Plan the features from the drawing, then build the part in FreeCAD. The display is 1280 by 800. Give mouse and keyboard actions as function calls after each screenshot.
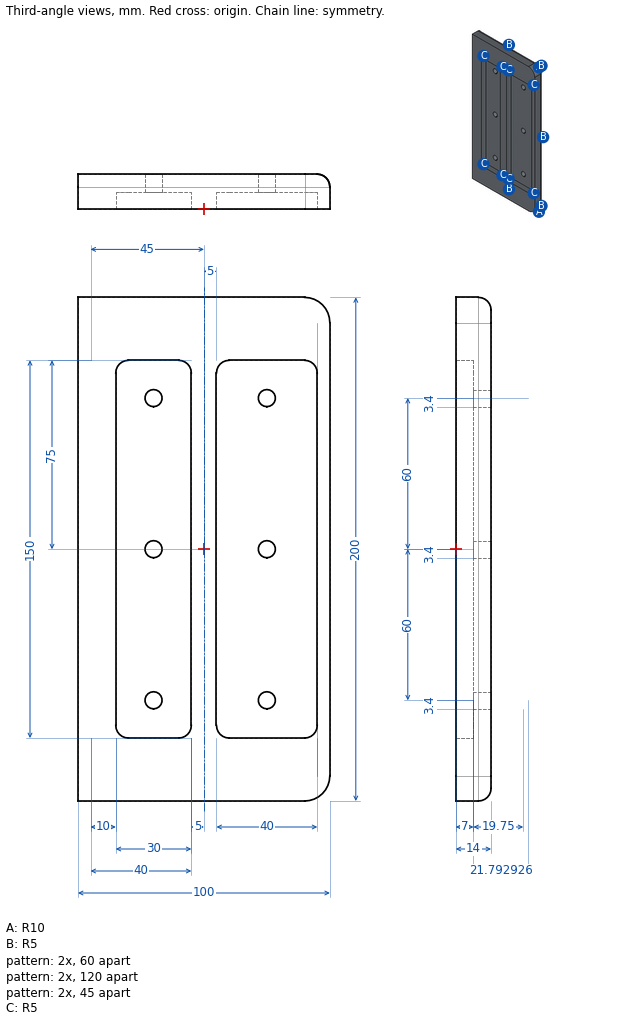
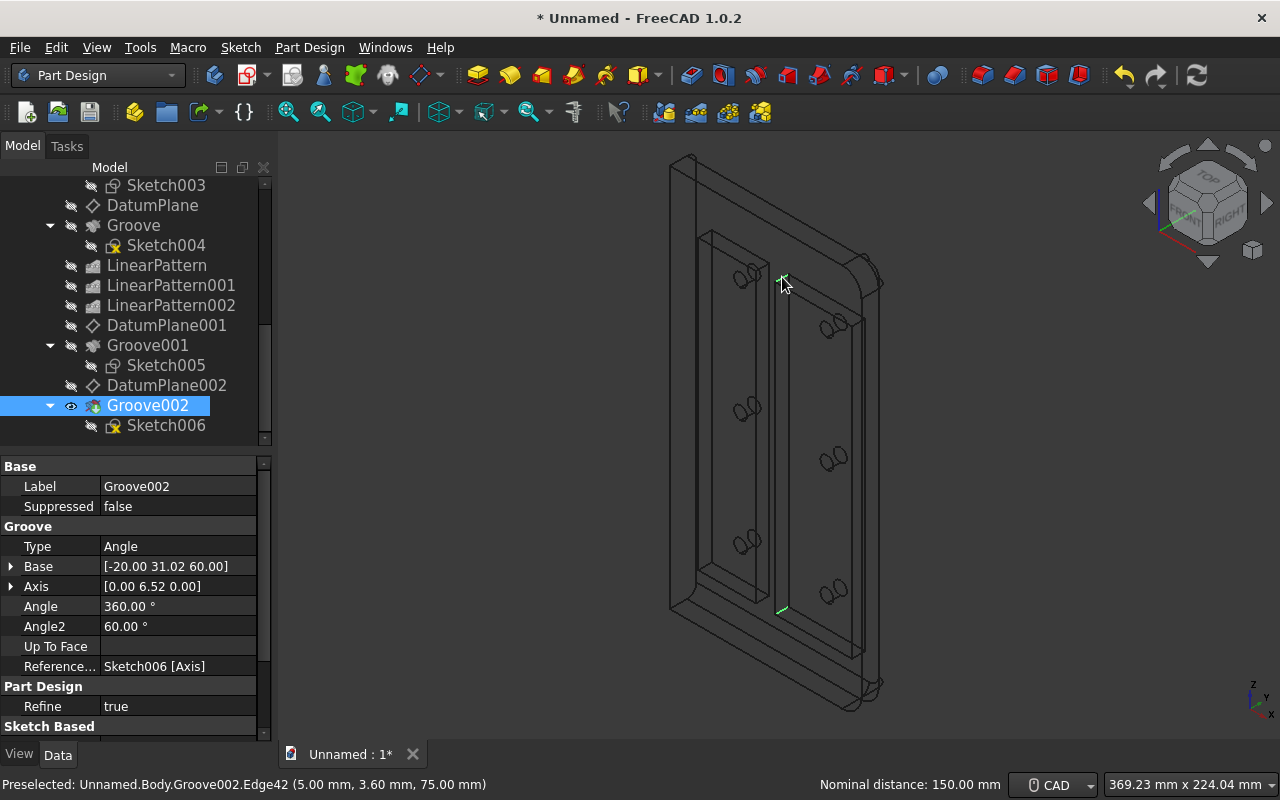
click(763, 266, ctrl)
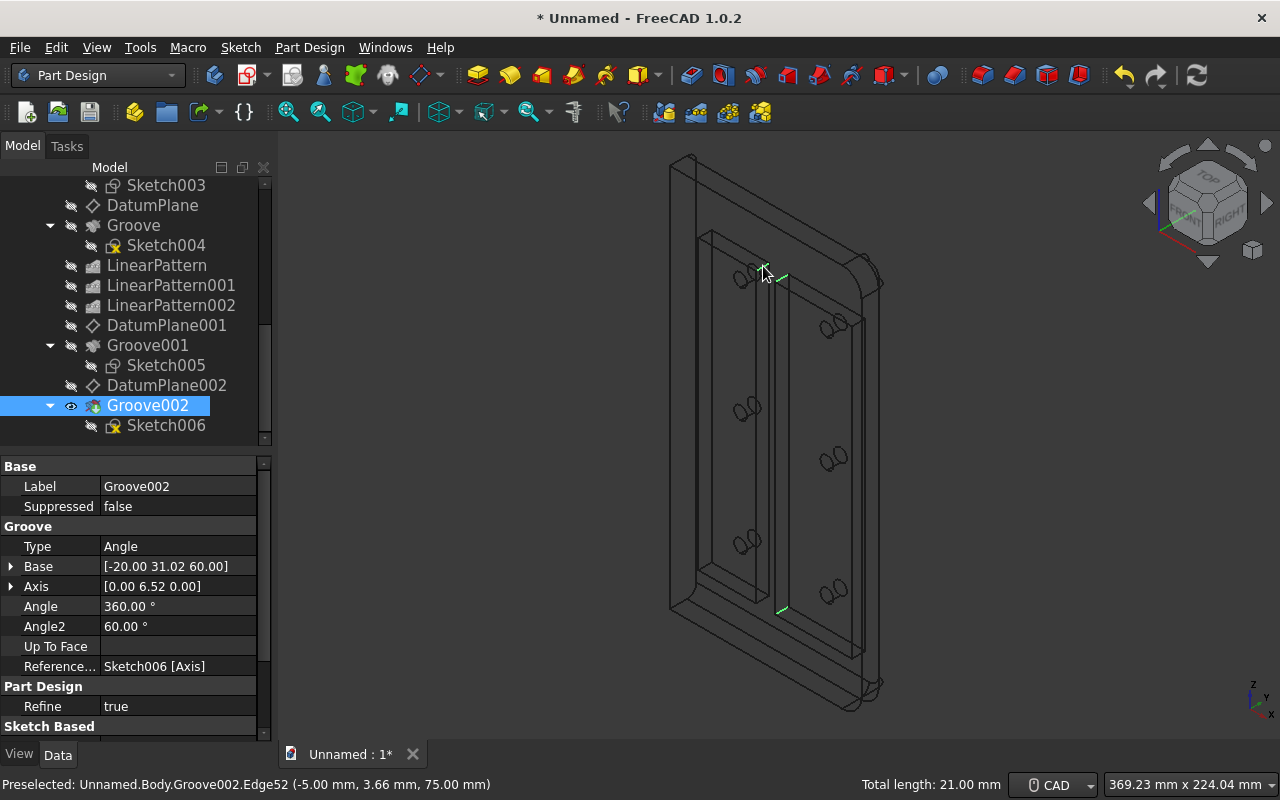
click(705, 565, ctrl)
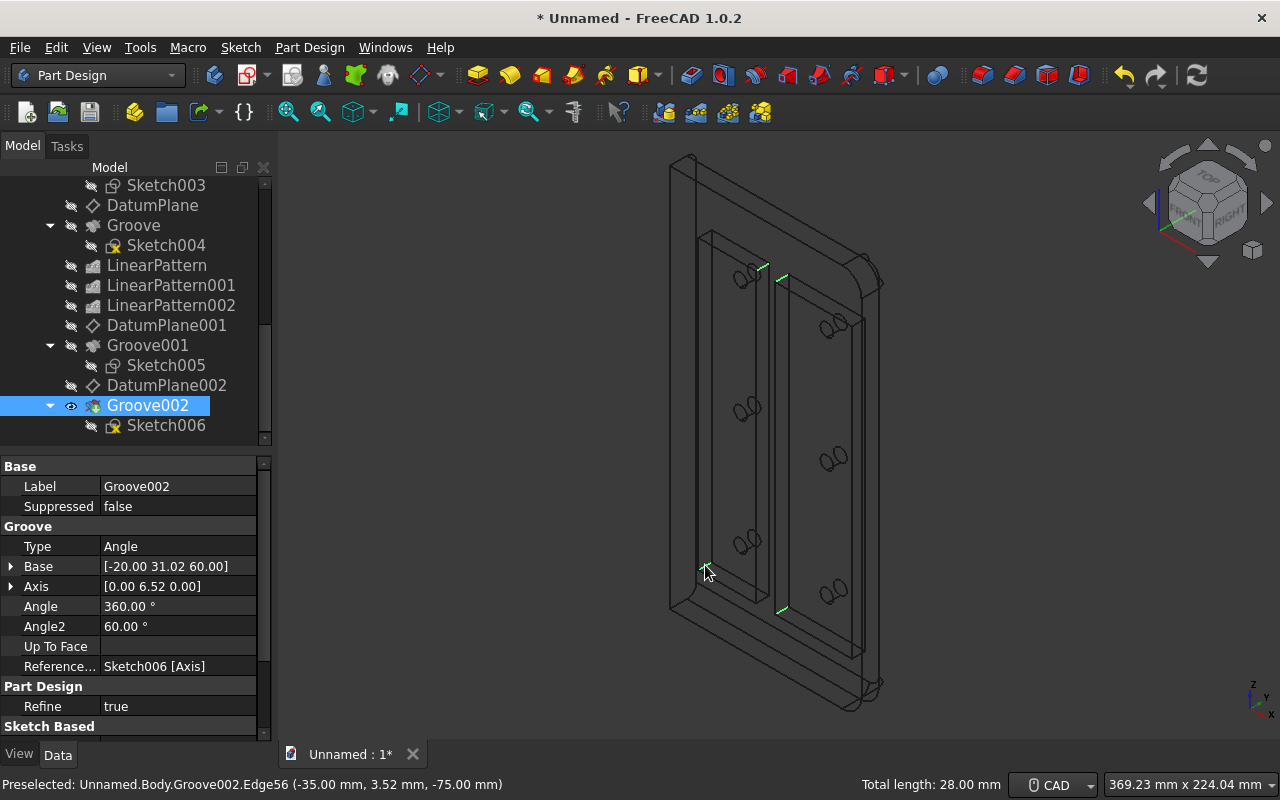
click(705, 233, ctrl)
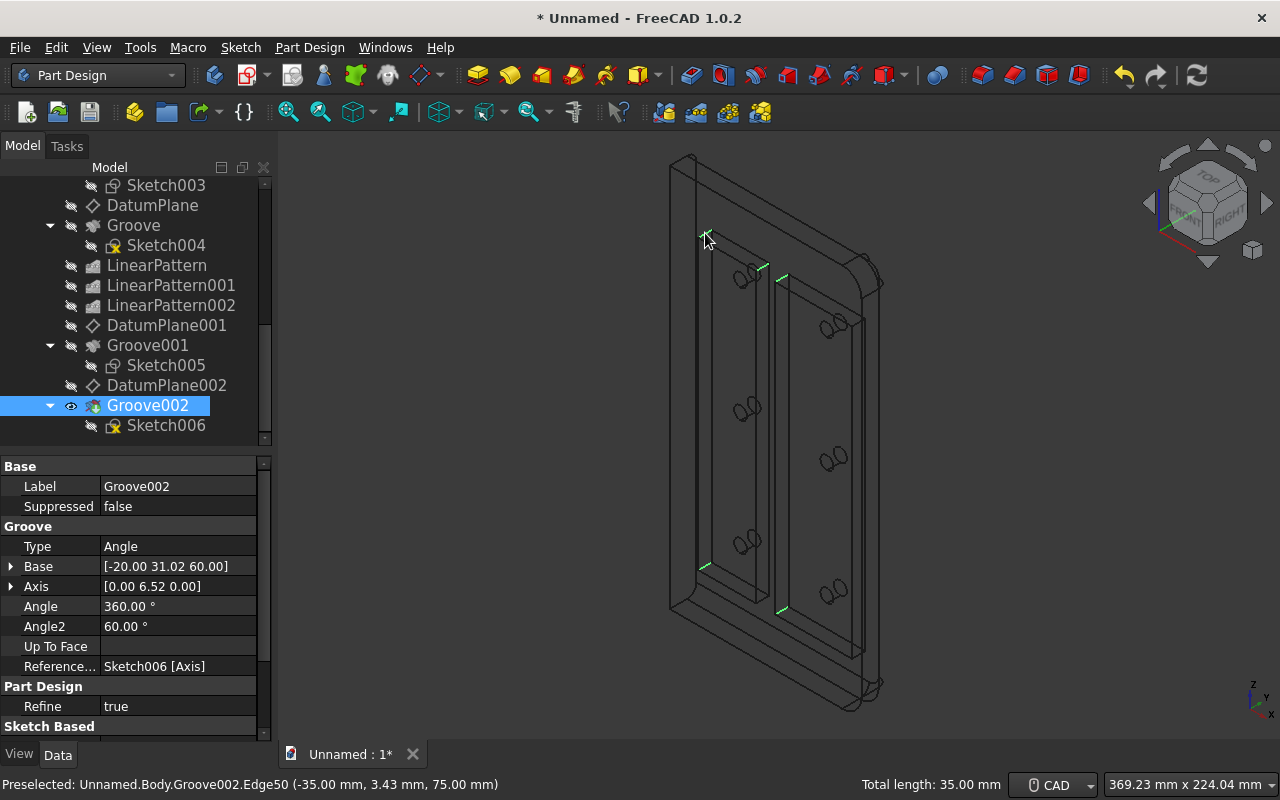
click(763, 599, ctrl)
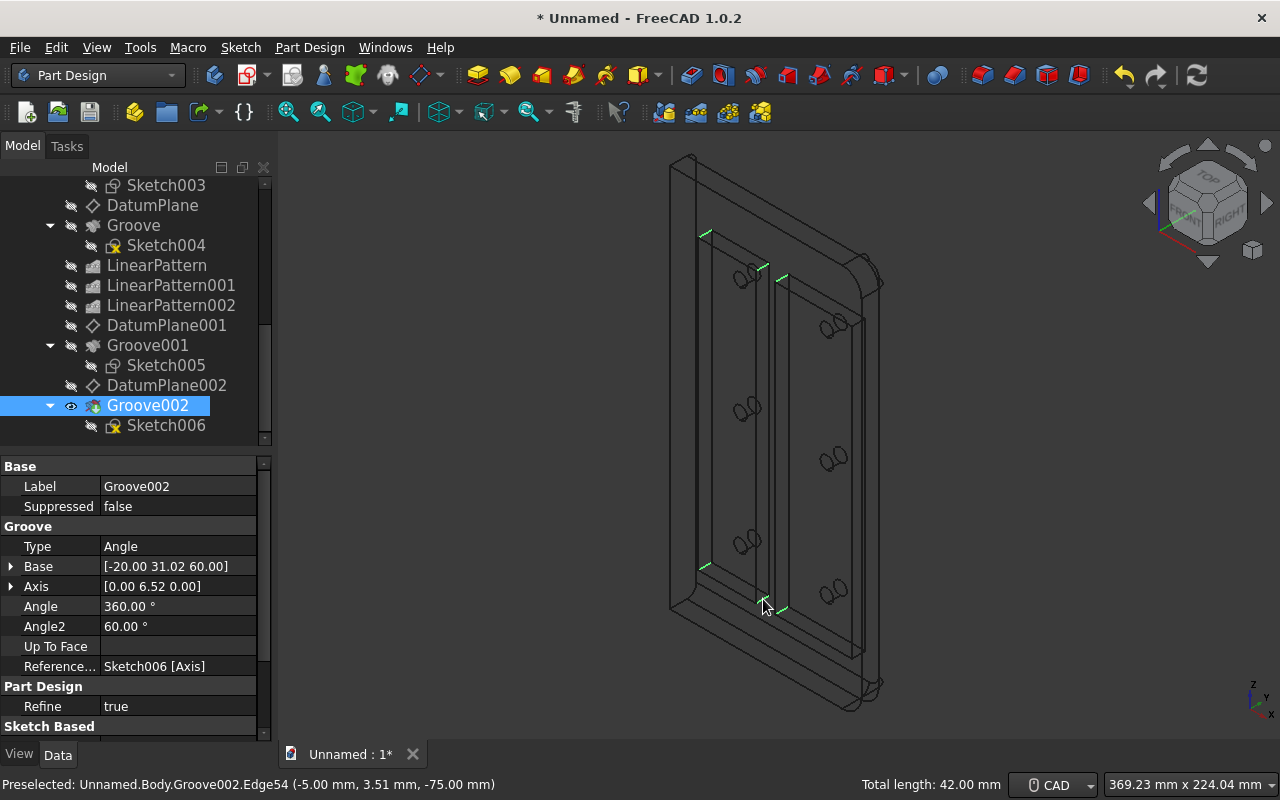
scroll(859, 322, up, 4)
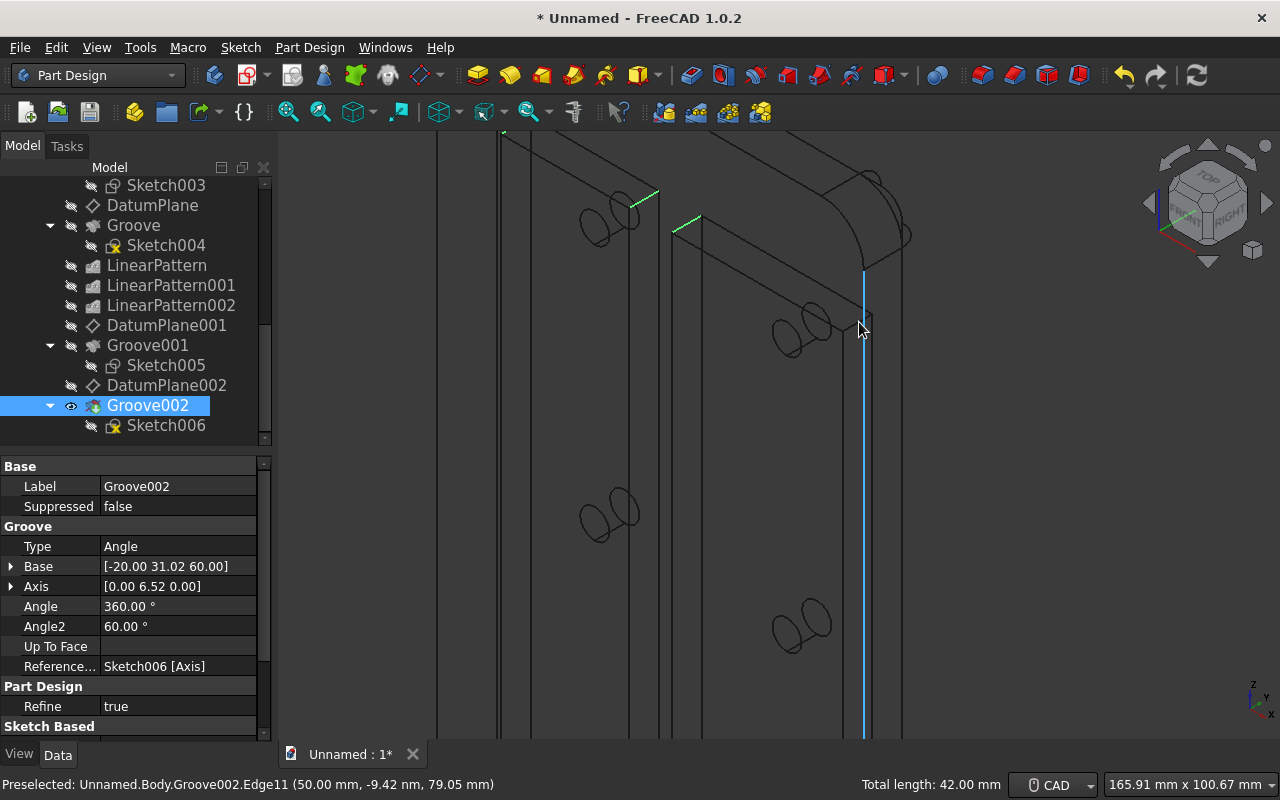
click(857, 322, ctrl)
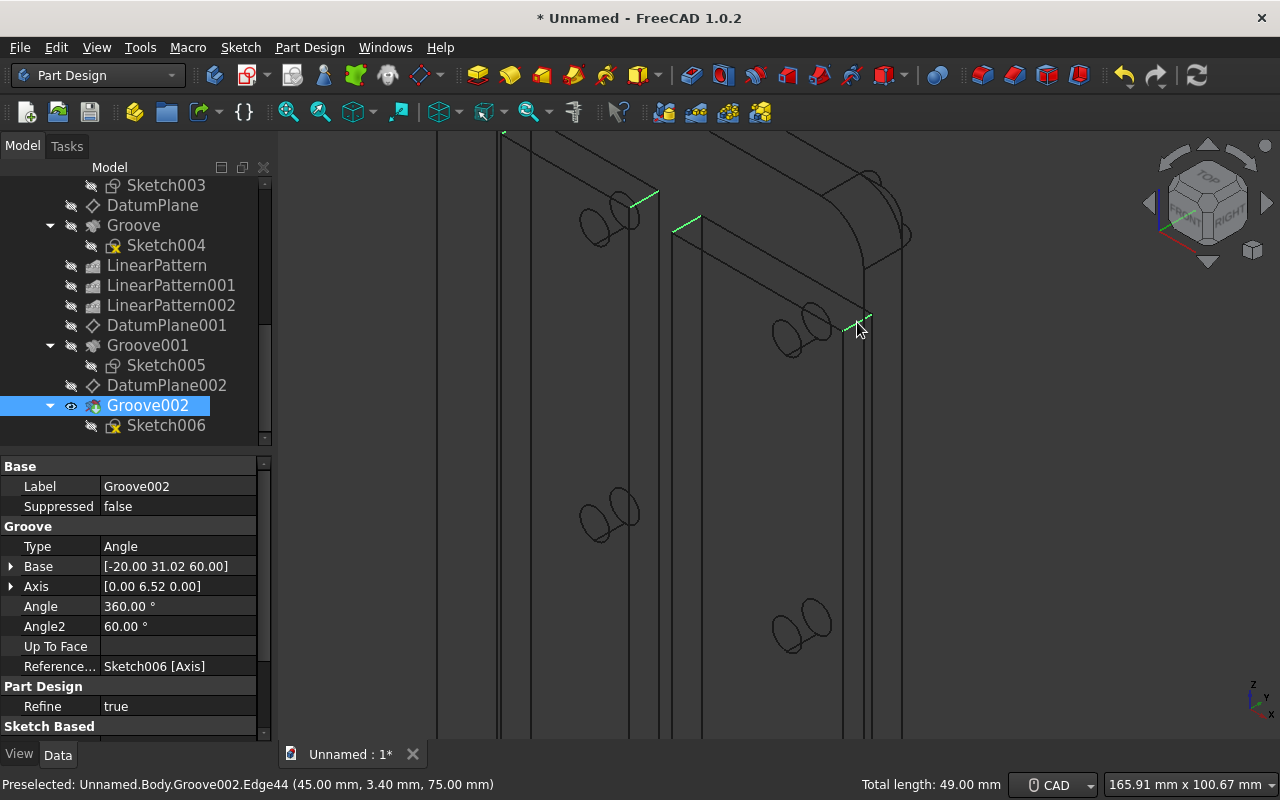
click(290, 112)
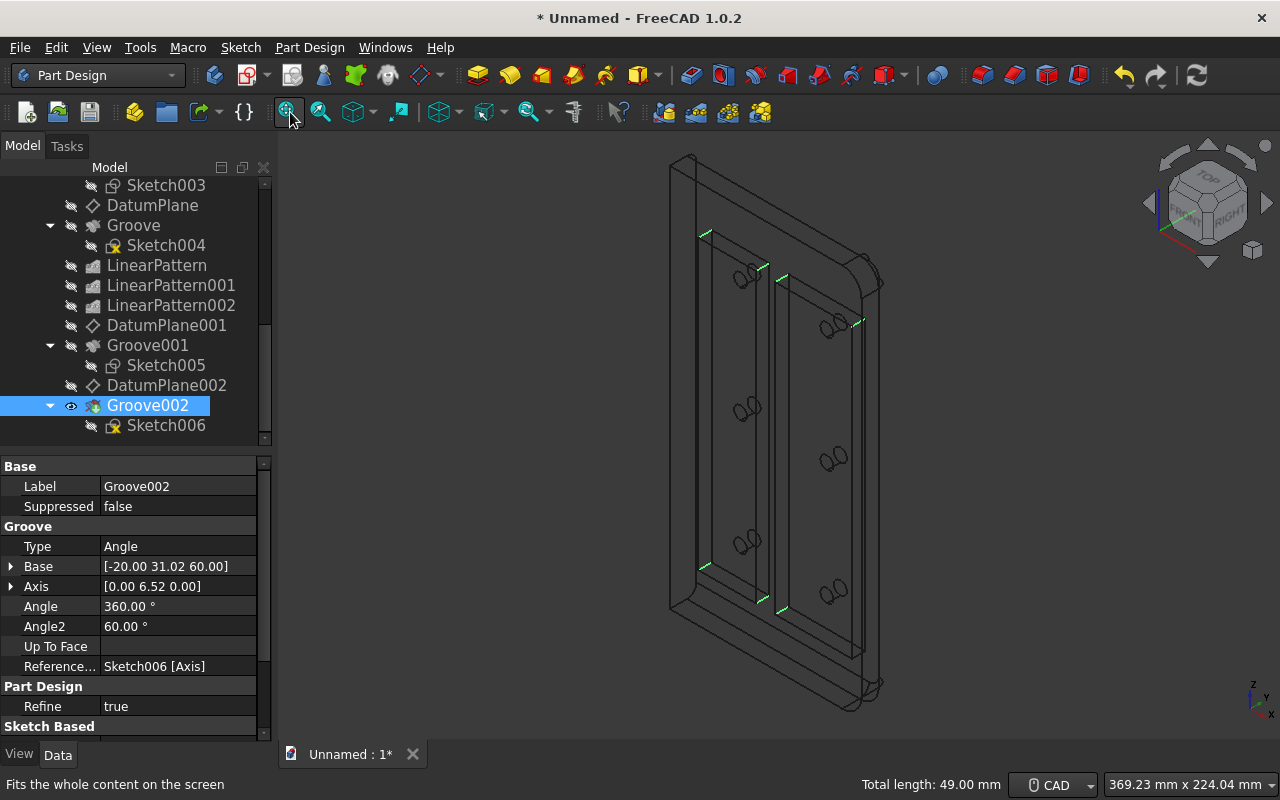
key(2)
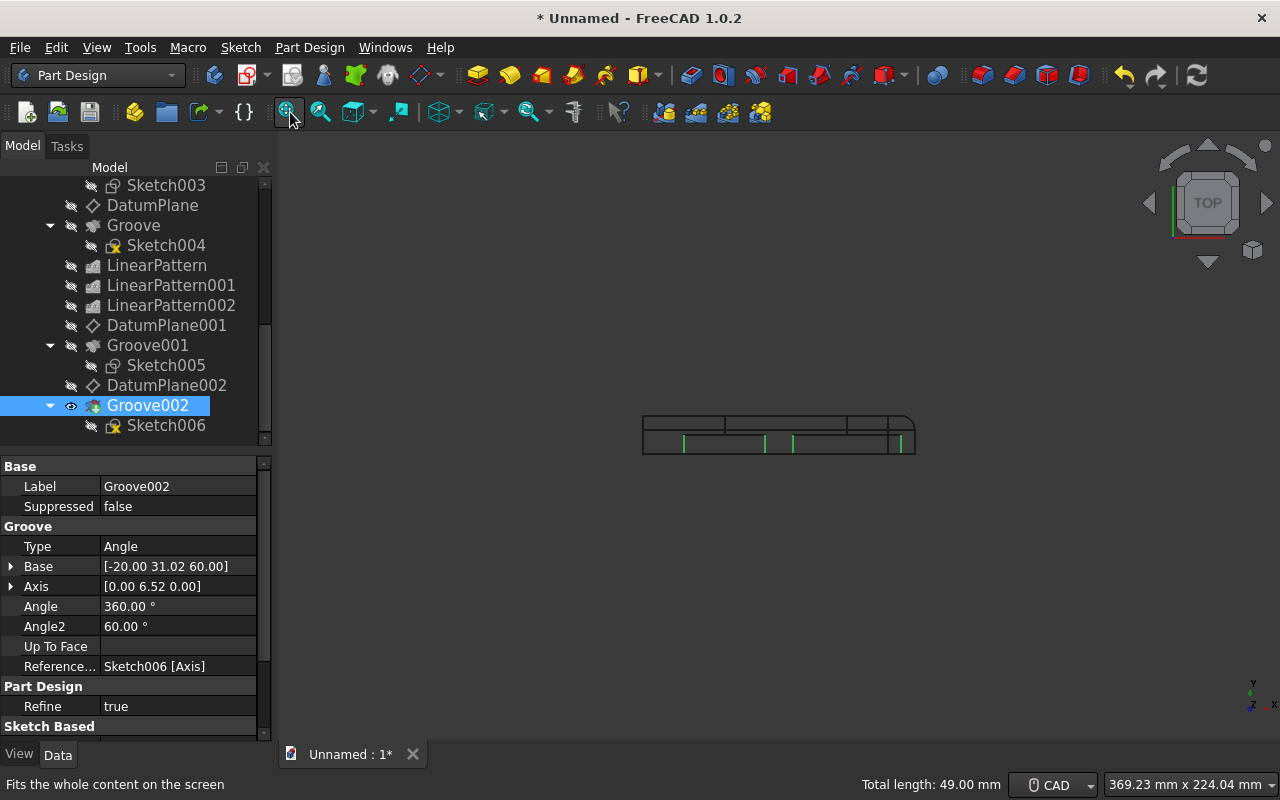
click(290, 112)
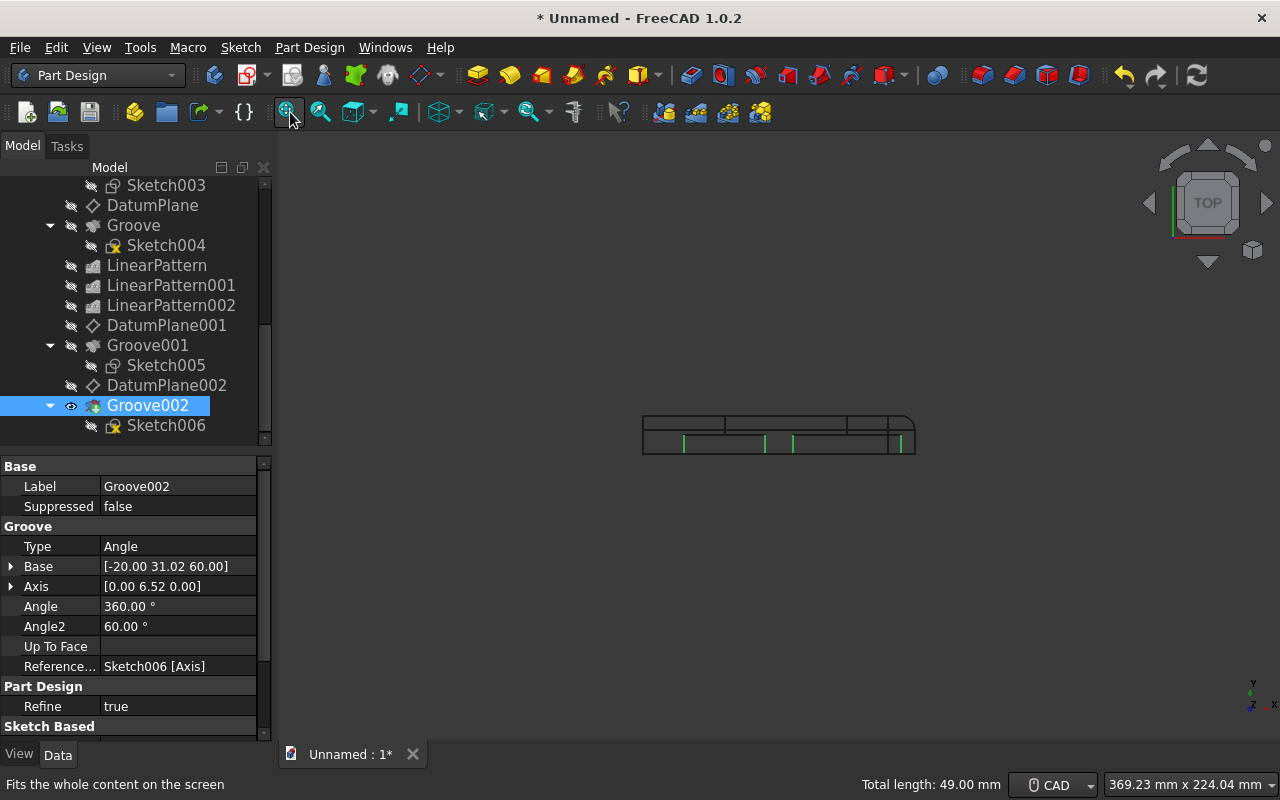
scroll(901, 443, up, 4)